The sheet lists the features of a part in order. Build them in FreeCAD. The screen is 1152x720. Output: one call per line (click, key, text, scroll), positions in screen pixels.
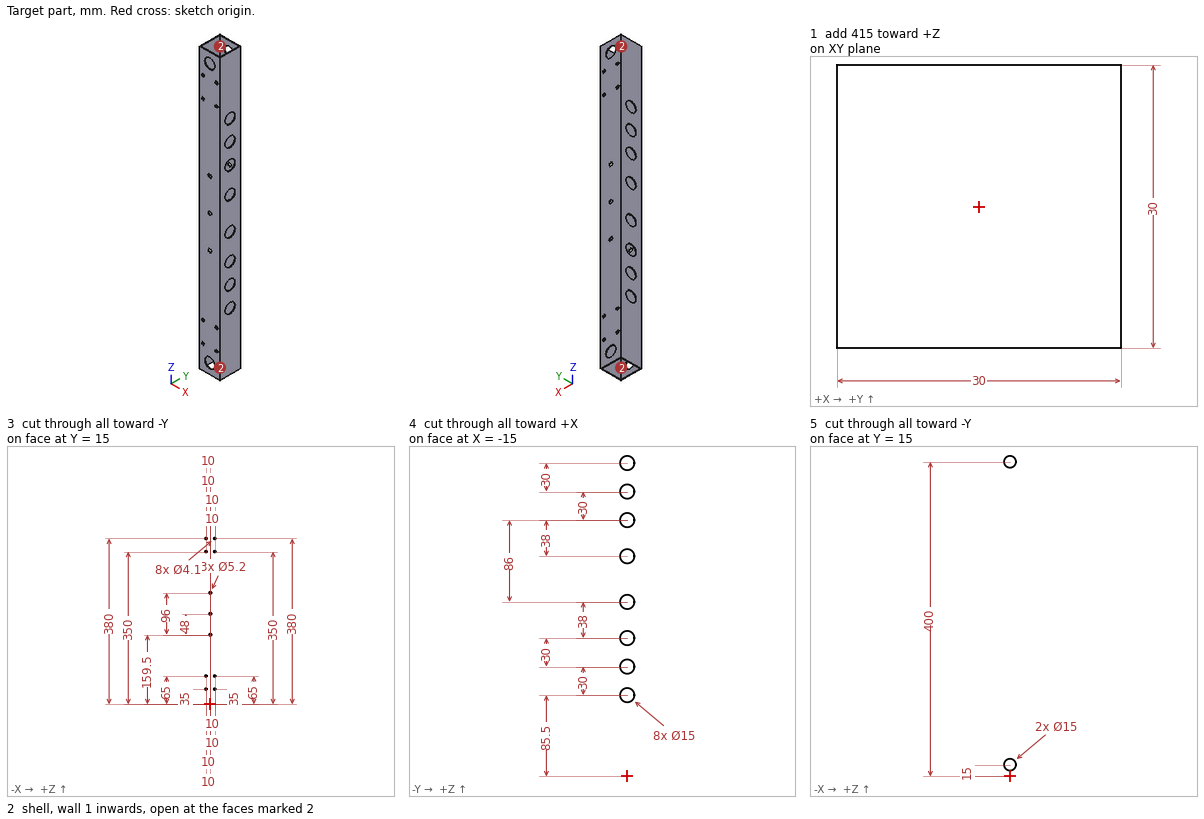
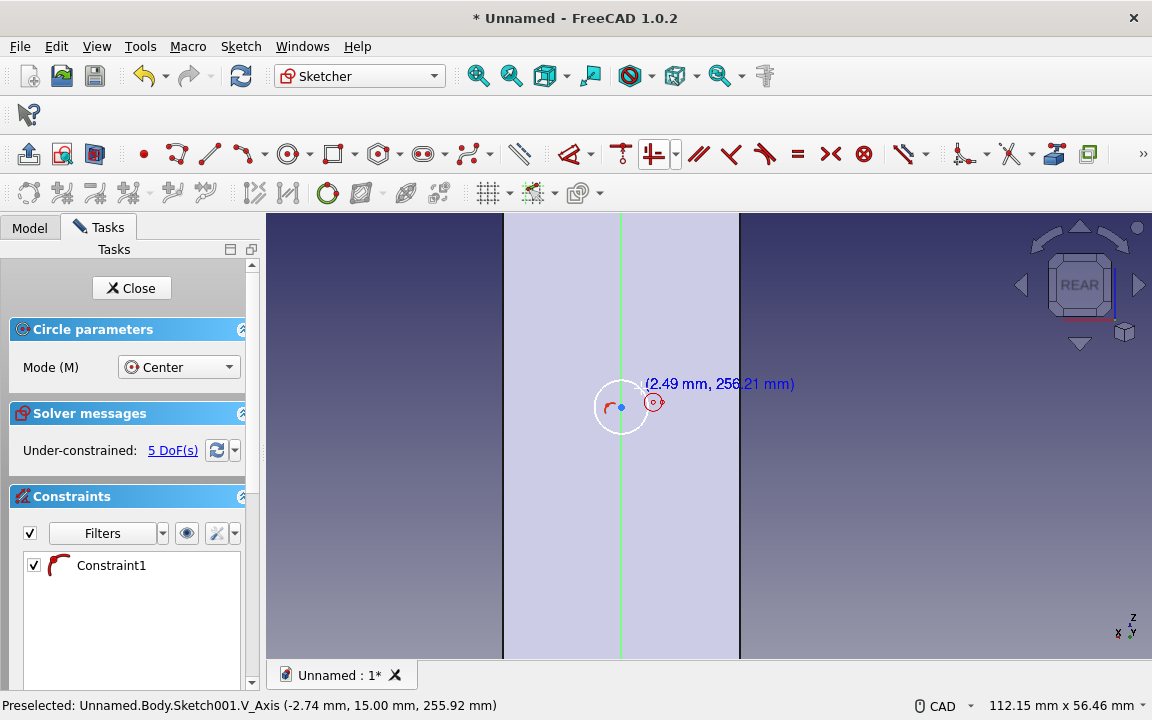
scroll(642, 389, down, 12)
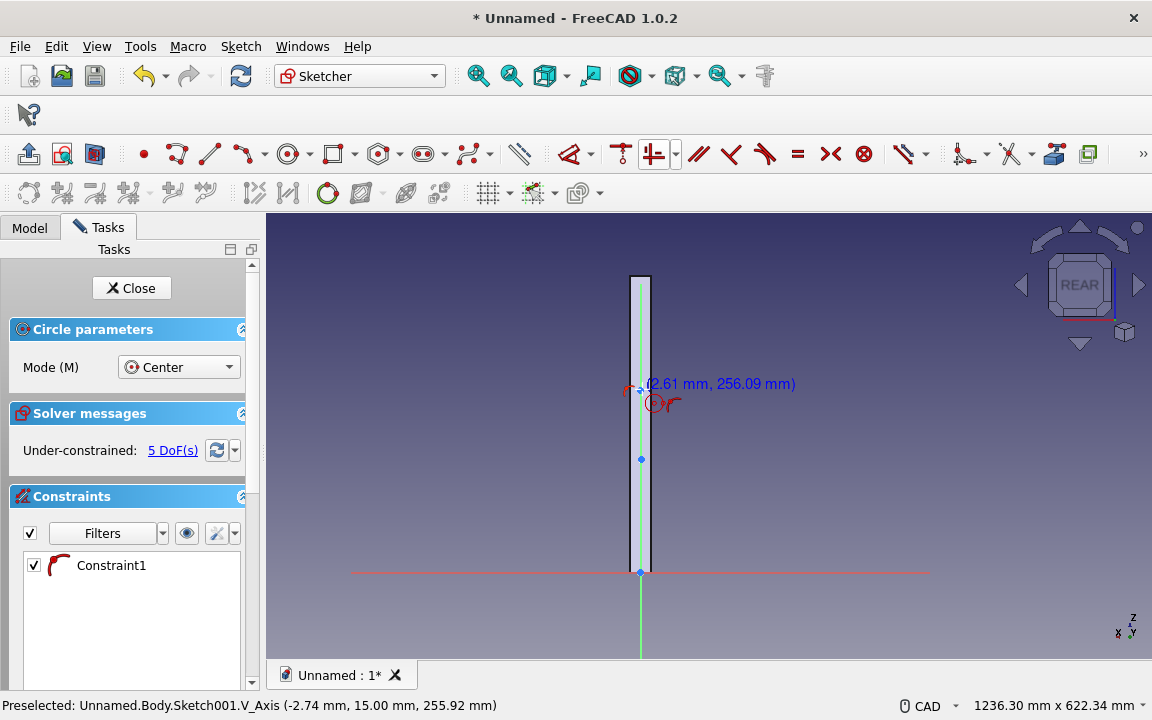
scroll(641, 424, up, 13)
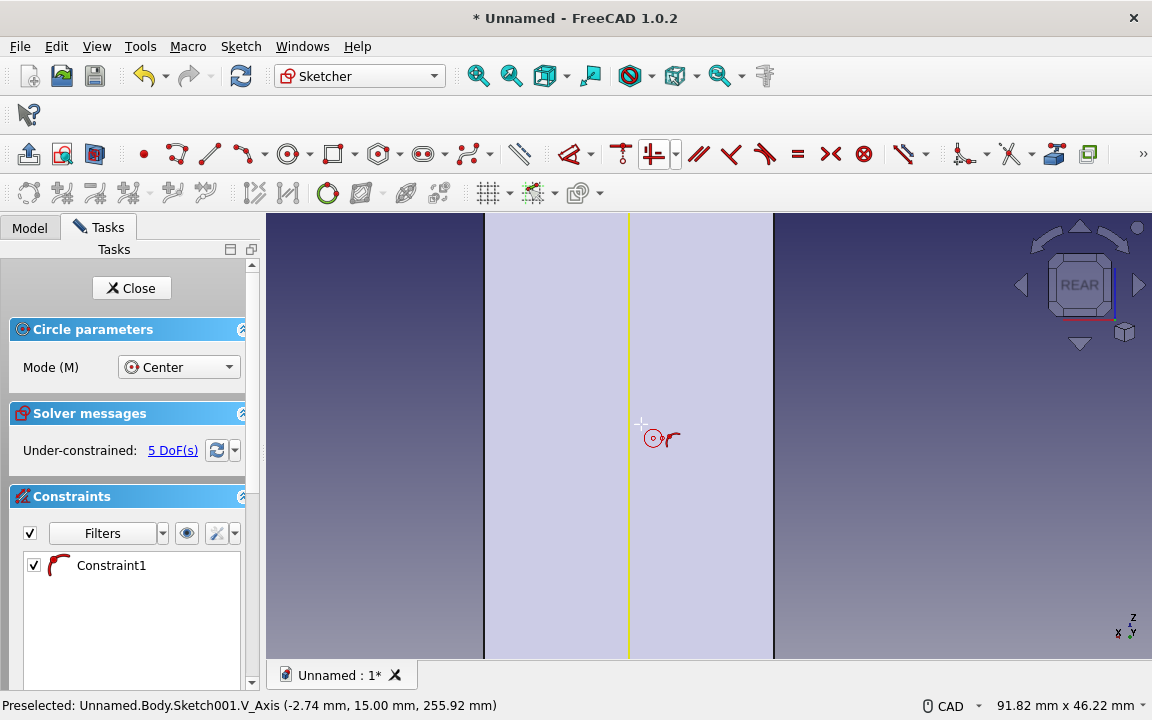
scroll(641, 424, down, 13)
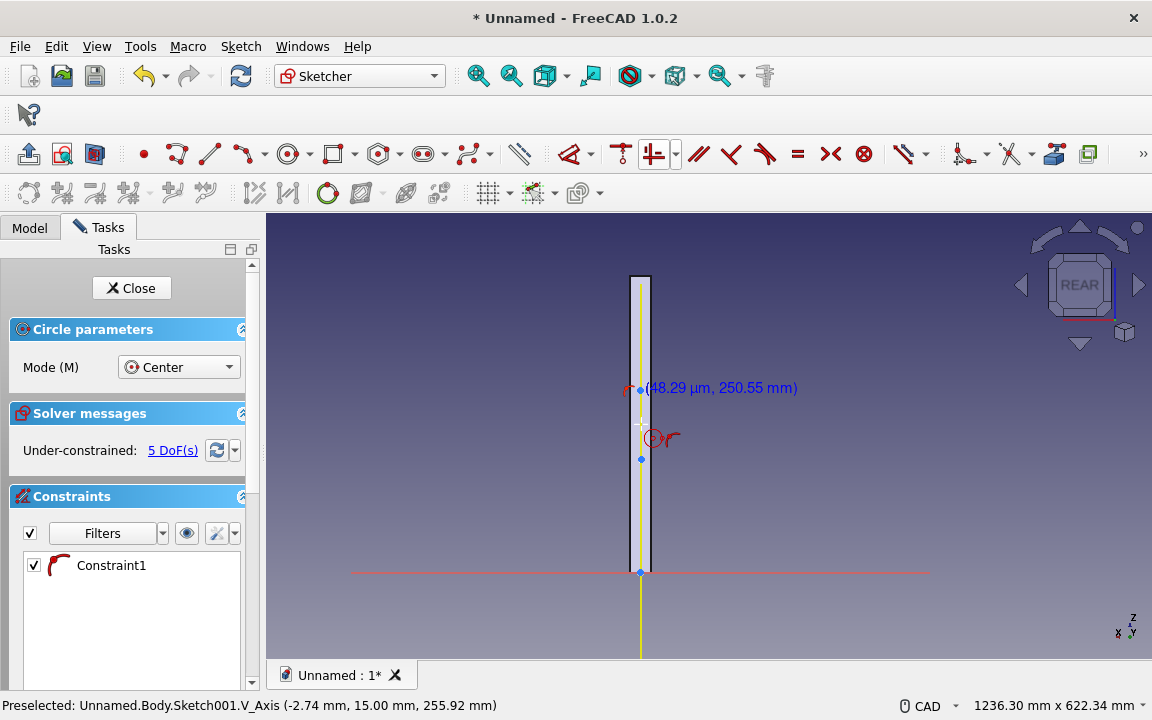
click(641, 424)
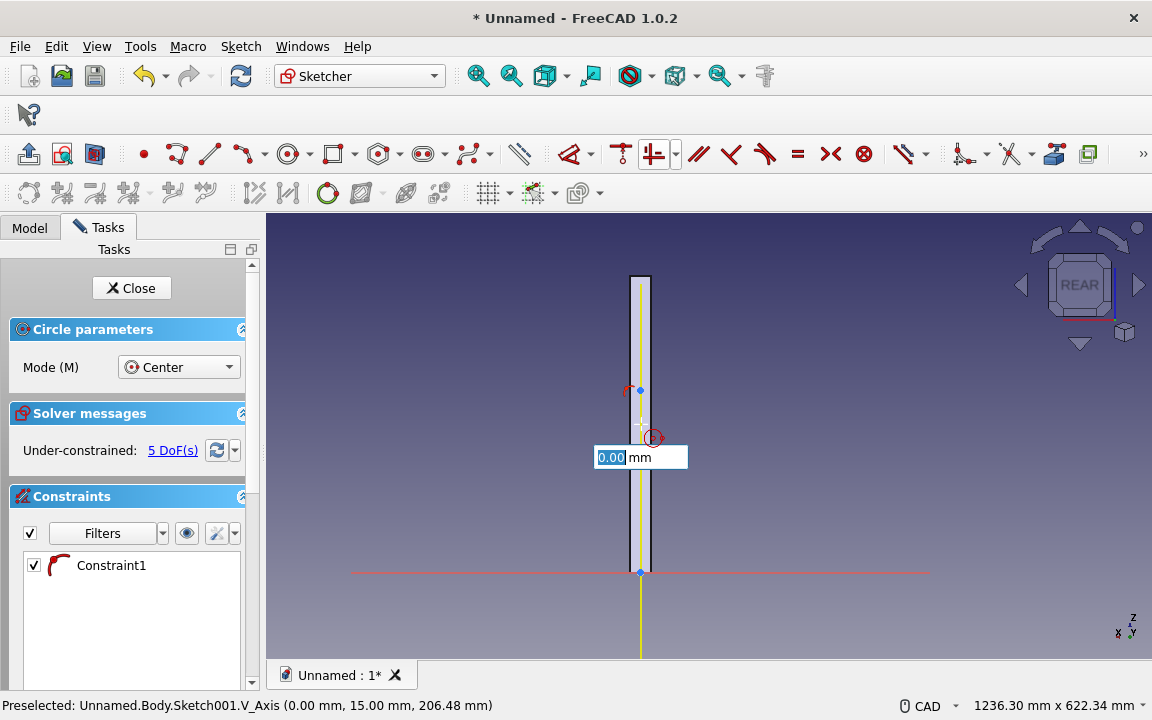
scroll(642, 424, up, 12)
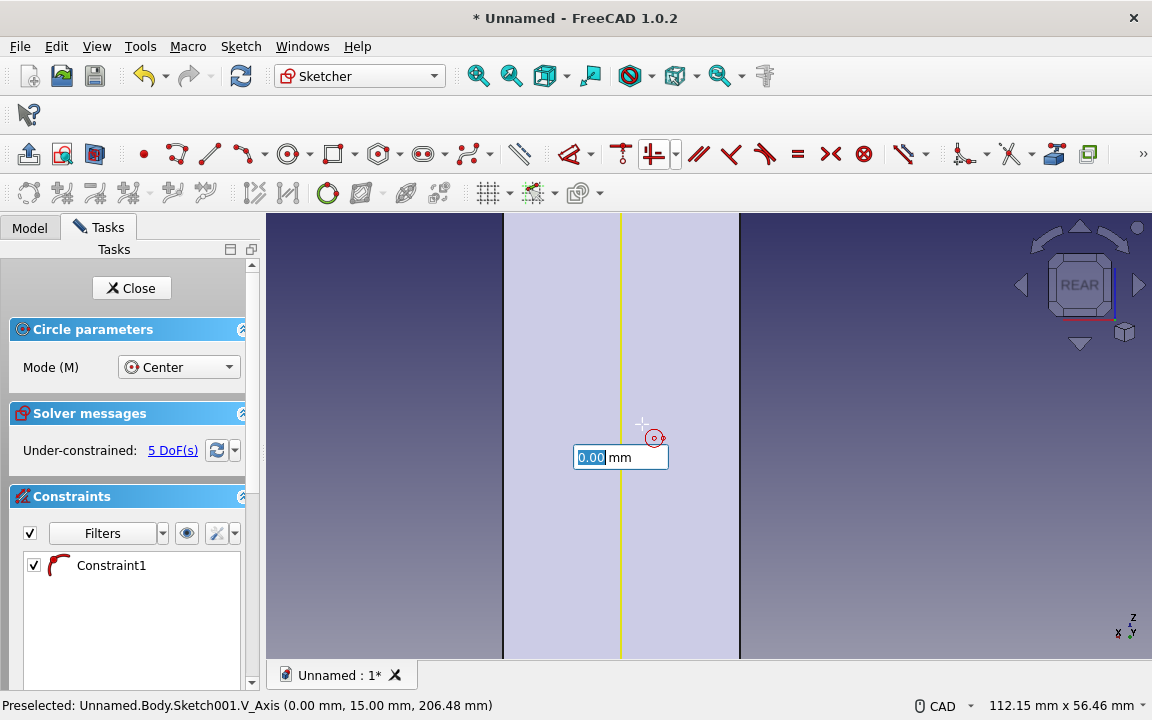
click(641, 415)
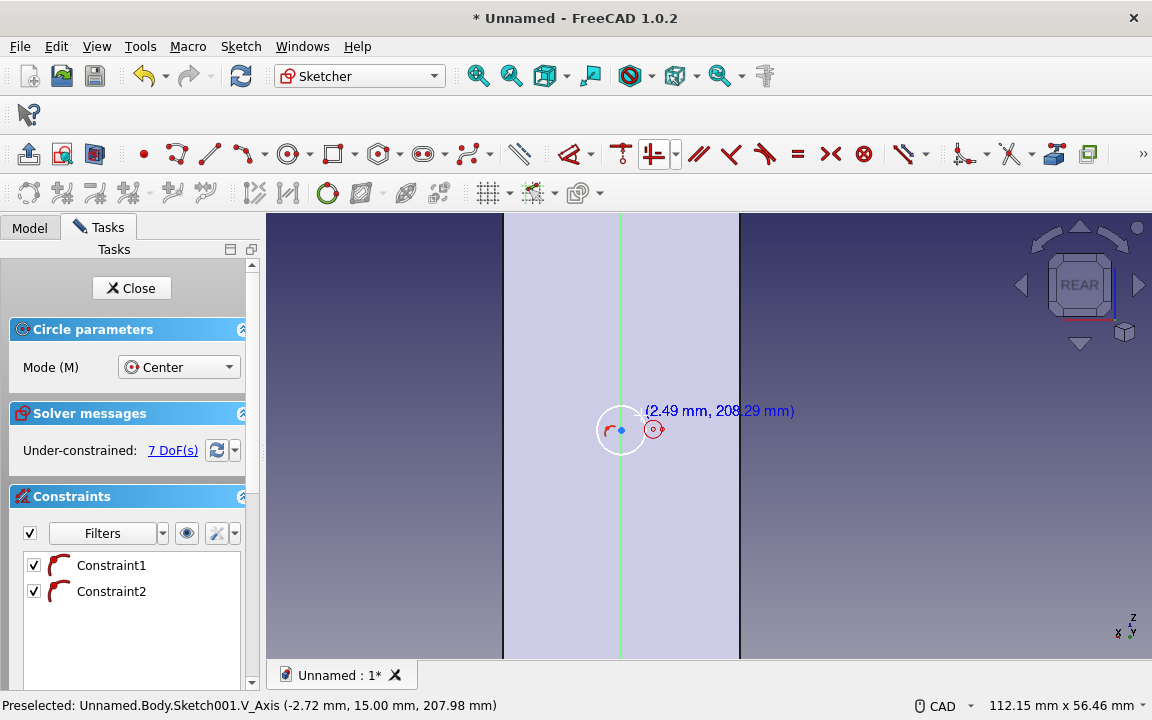
scroll(642, 424, down, 12)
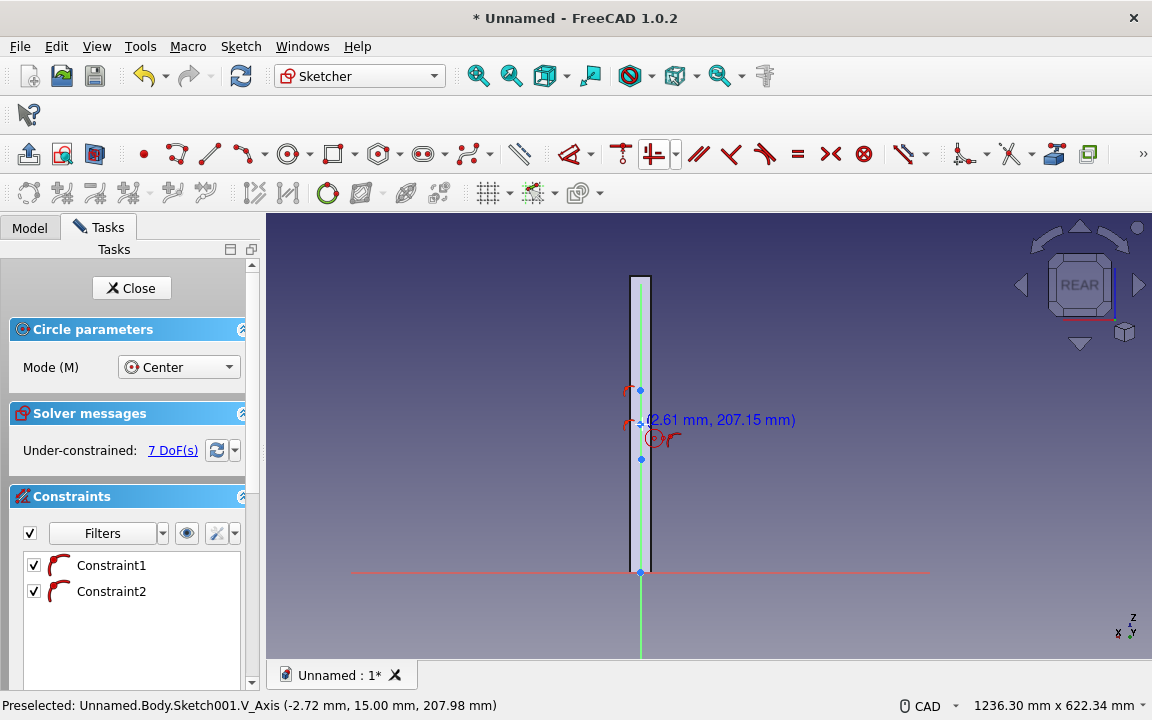
scroll(648, 548, up, 14)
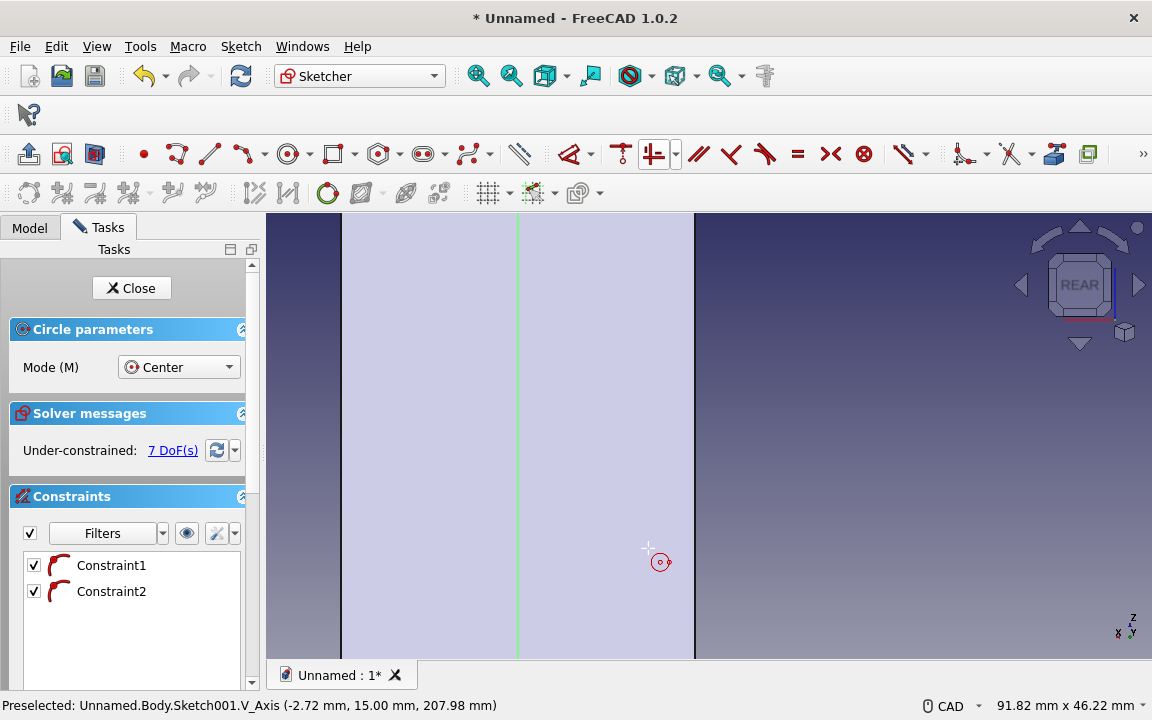
scroll(648, 549, down, 14)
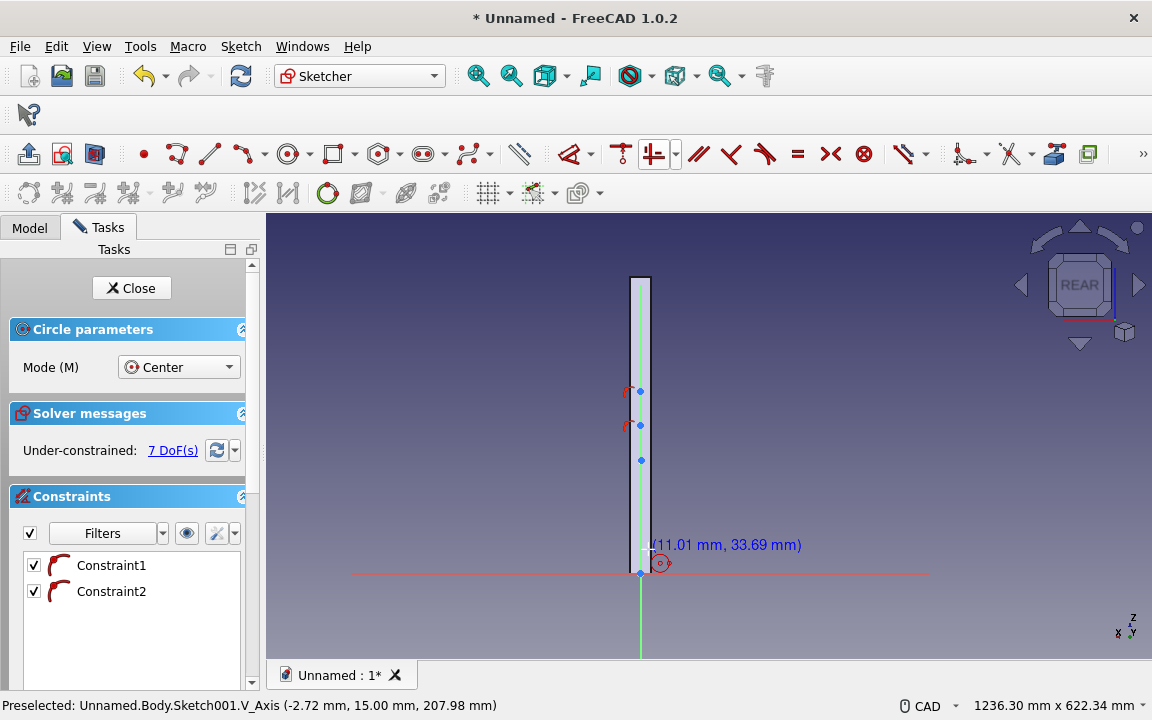
scroll(648, 549, up, 4)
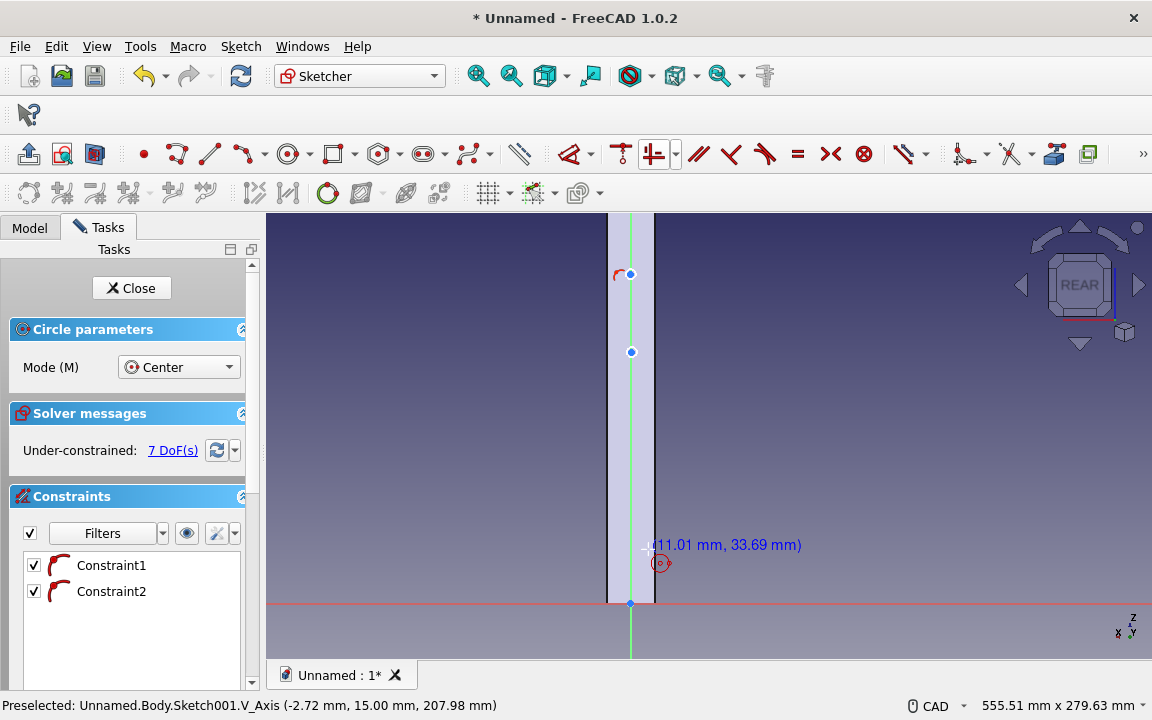
click(647, 548)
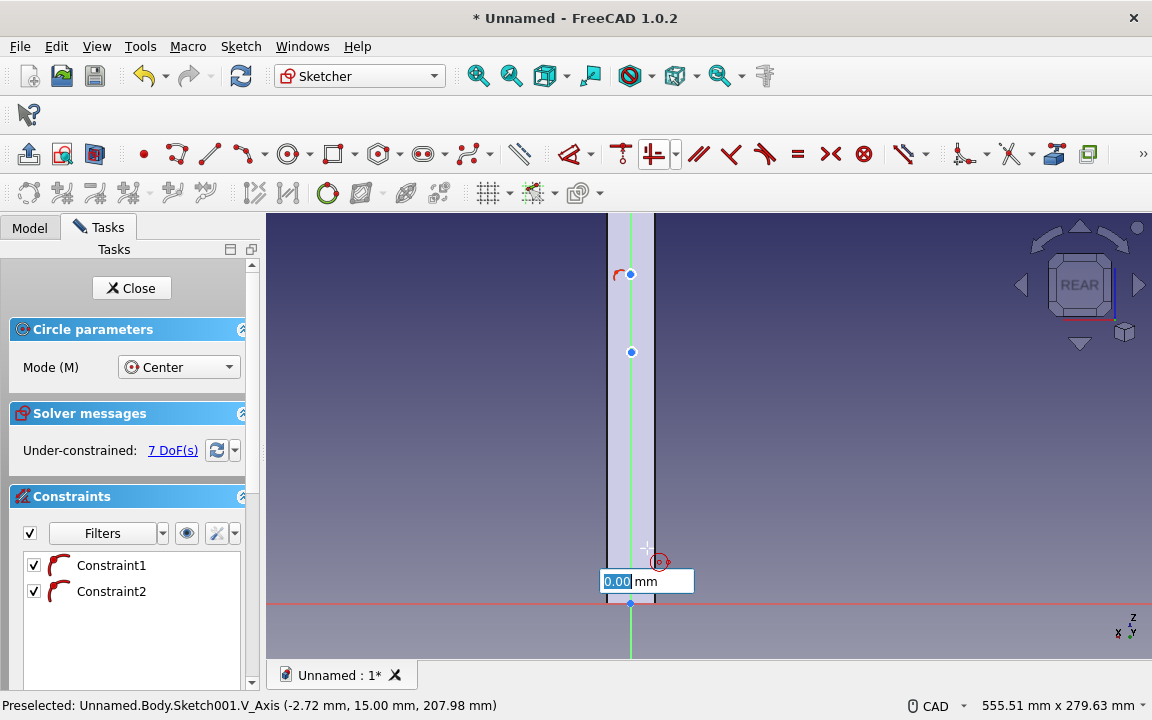
scroll(649, 545, up, 8)